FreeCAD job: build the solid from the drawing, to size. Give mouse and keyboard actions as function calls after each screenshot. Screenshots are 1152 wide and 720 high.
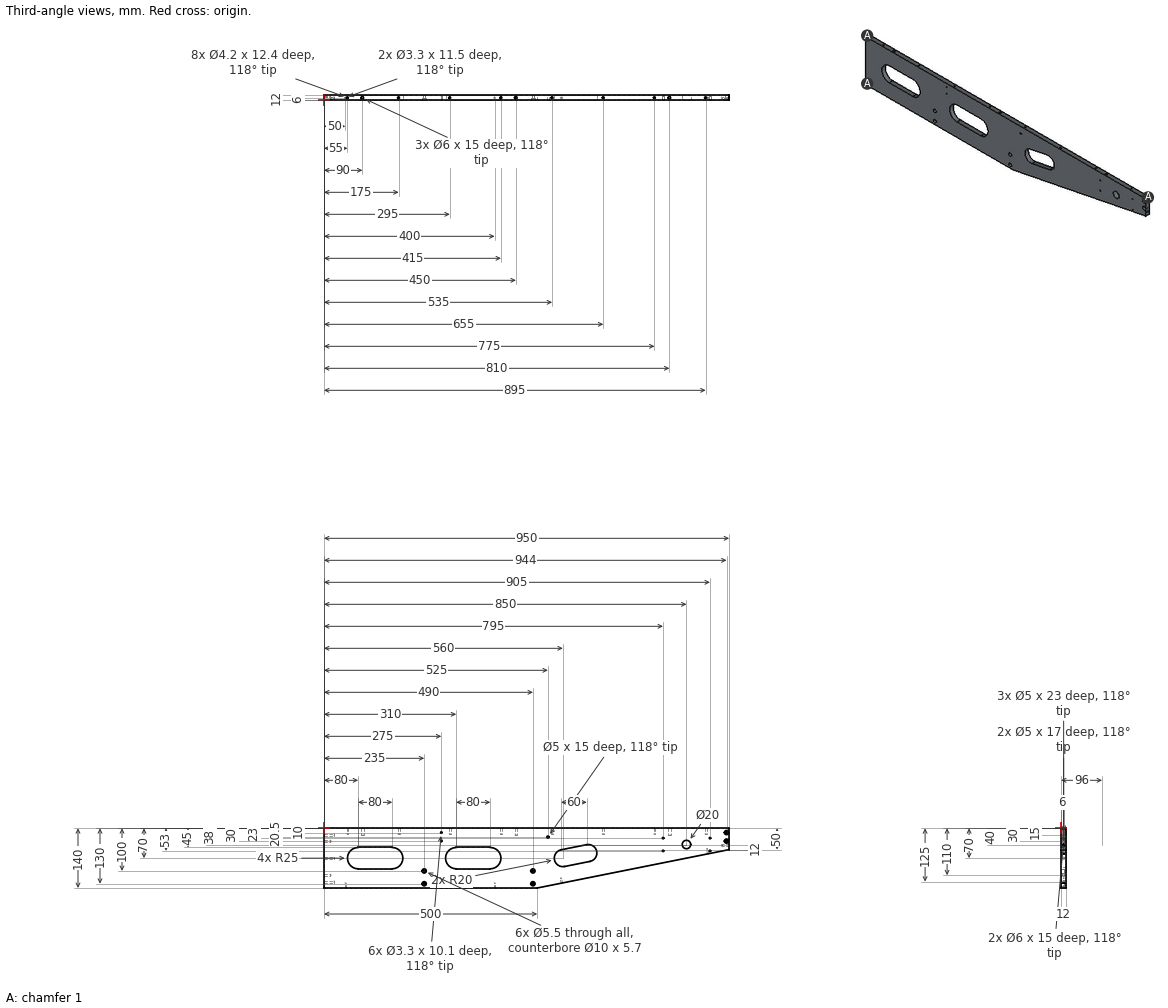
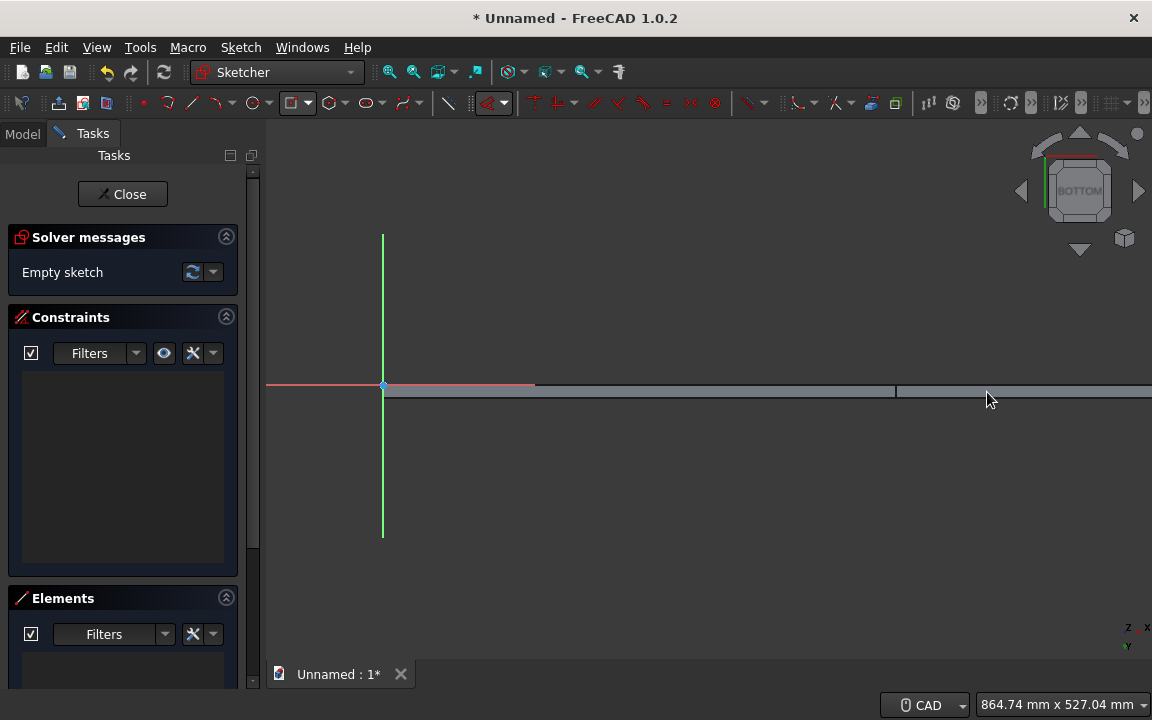
key(g)
key(c)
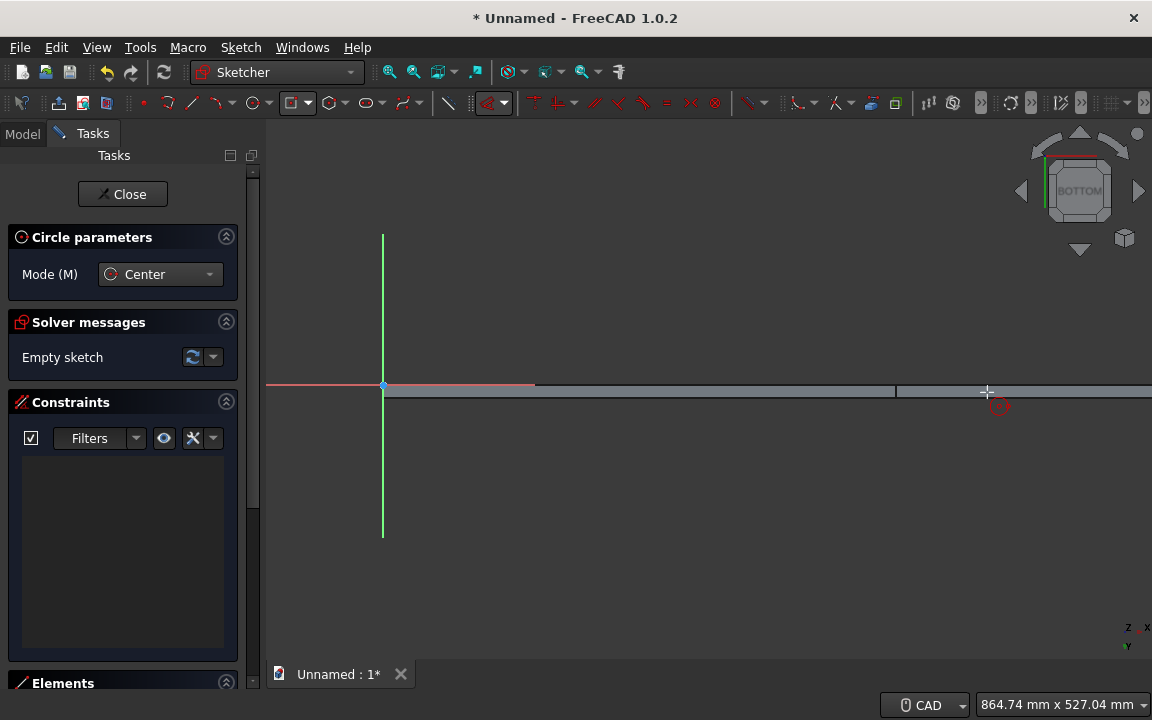
scroll(435, 392, up, 13)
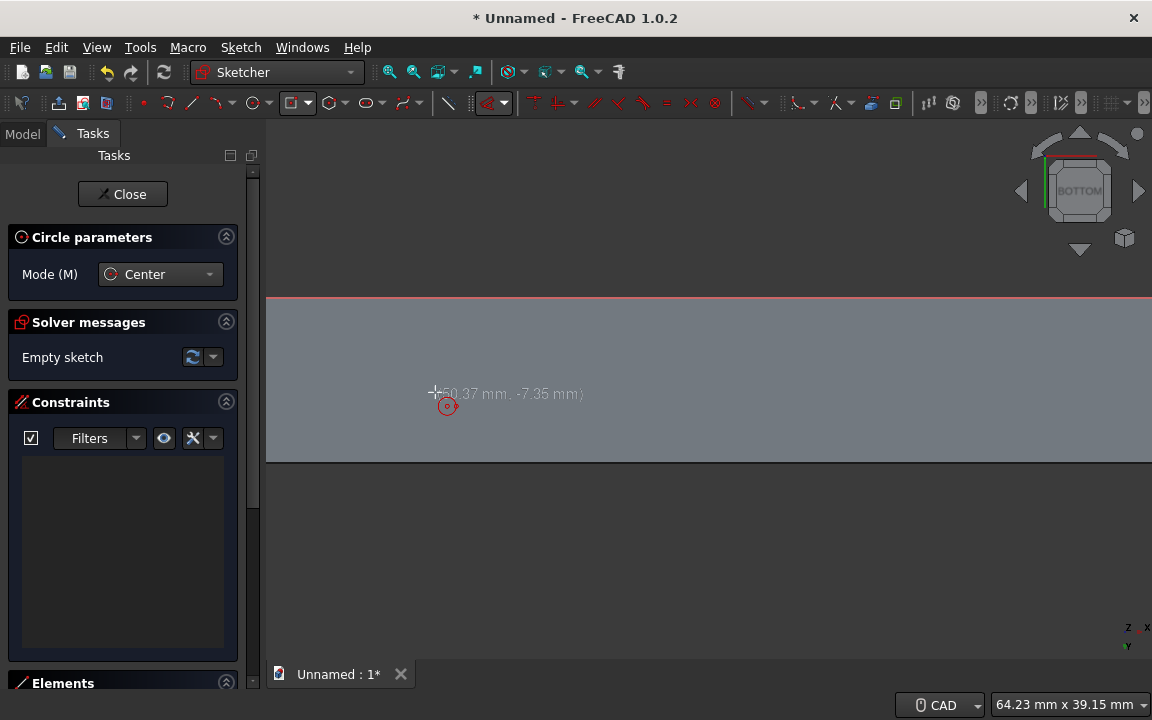
scroll(454, 393, down, 12)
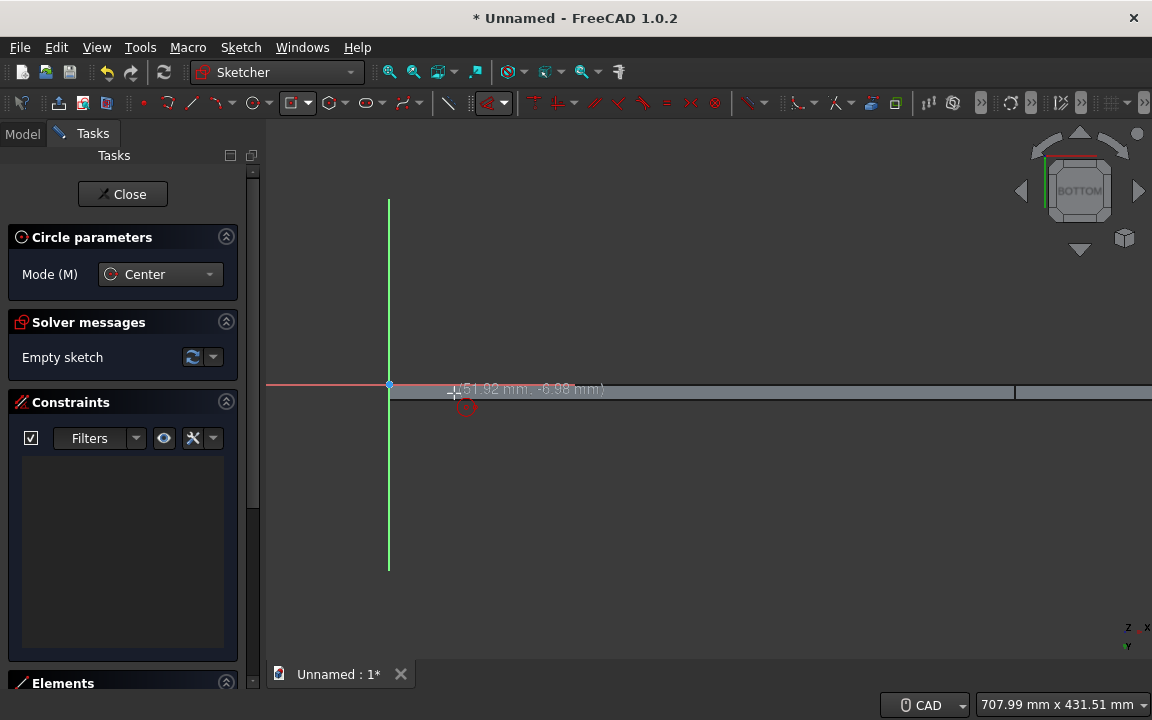
scroll(452, 392, up, 4)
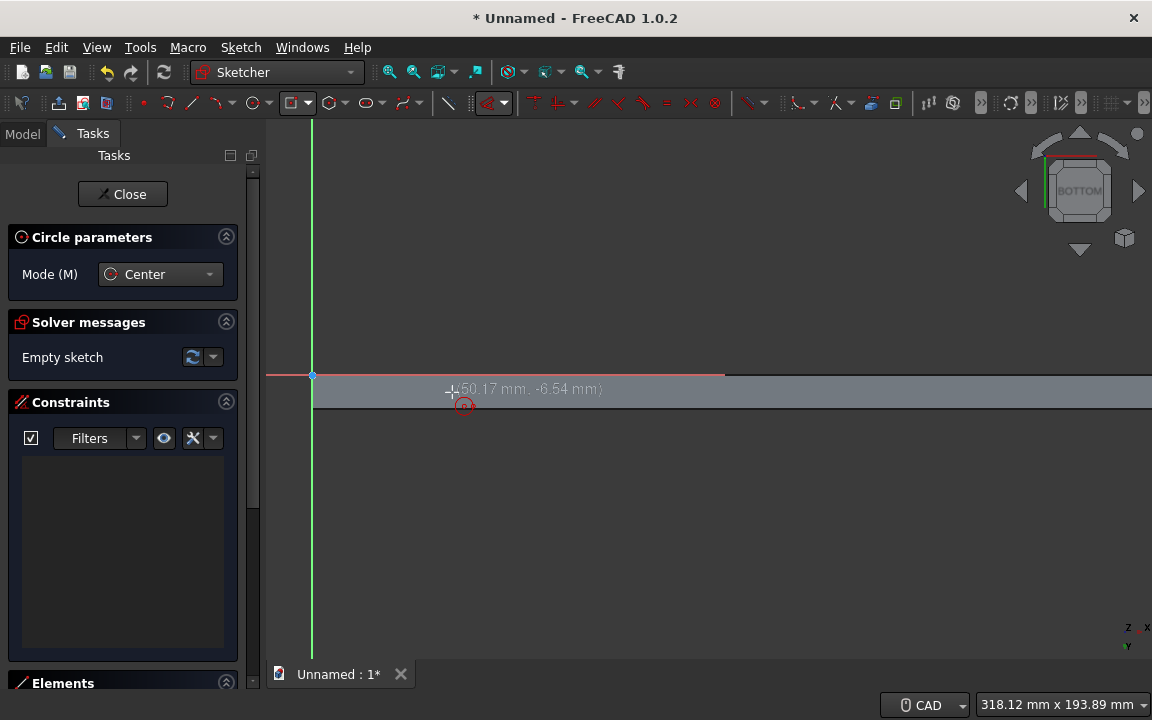
click(451, 392)
move(455, 395)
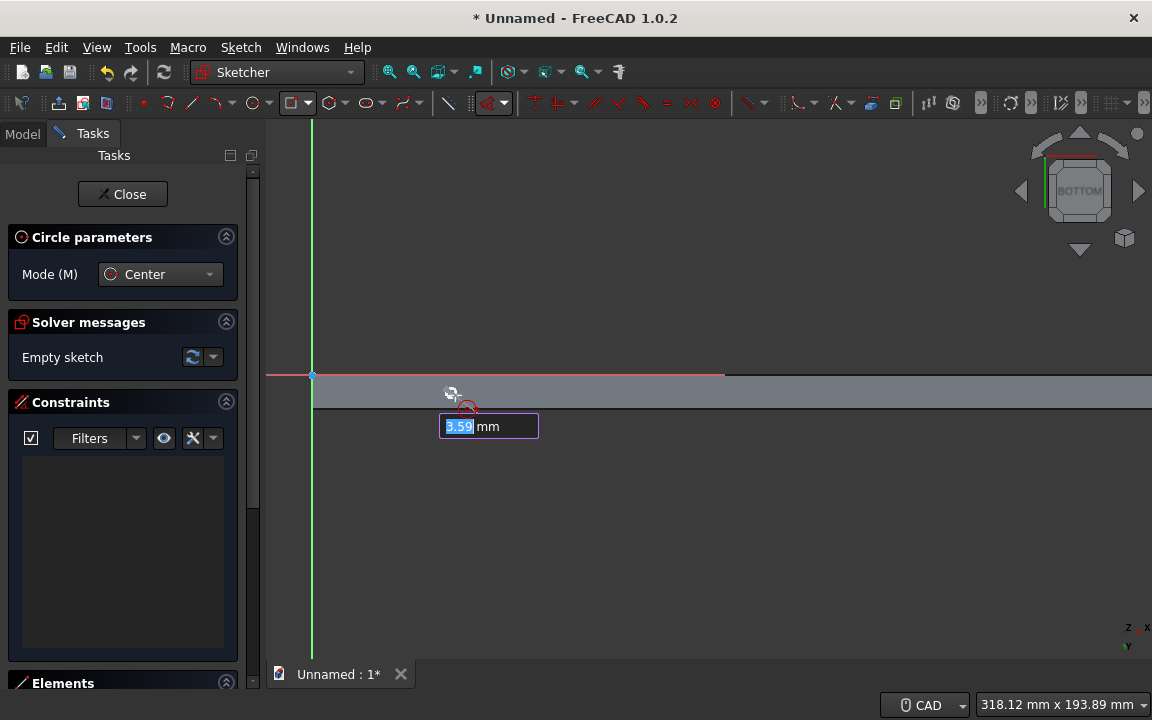
text(3.3)
key(Return)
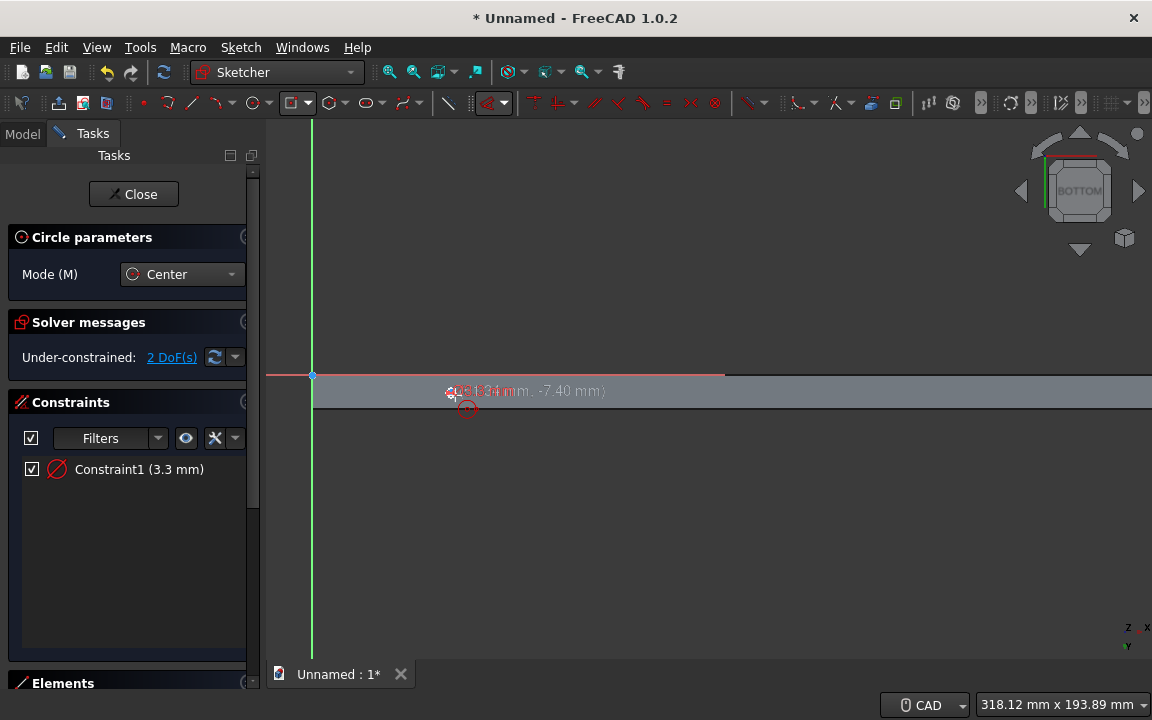
scroll(452, 391, down, 4)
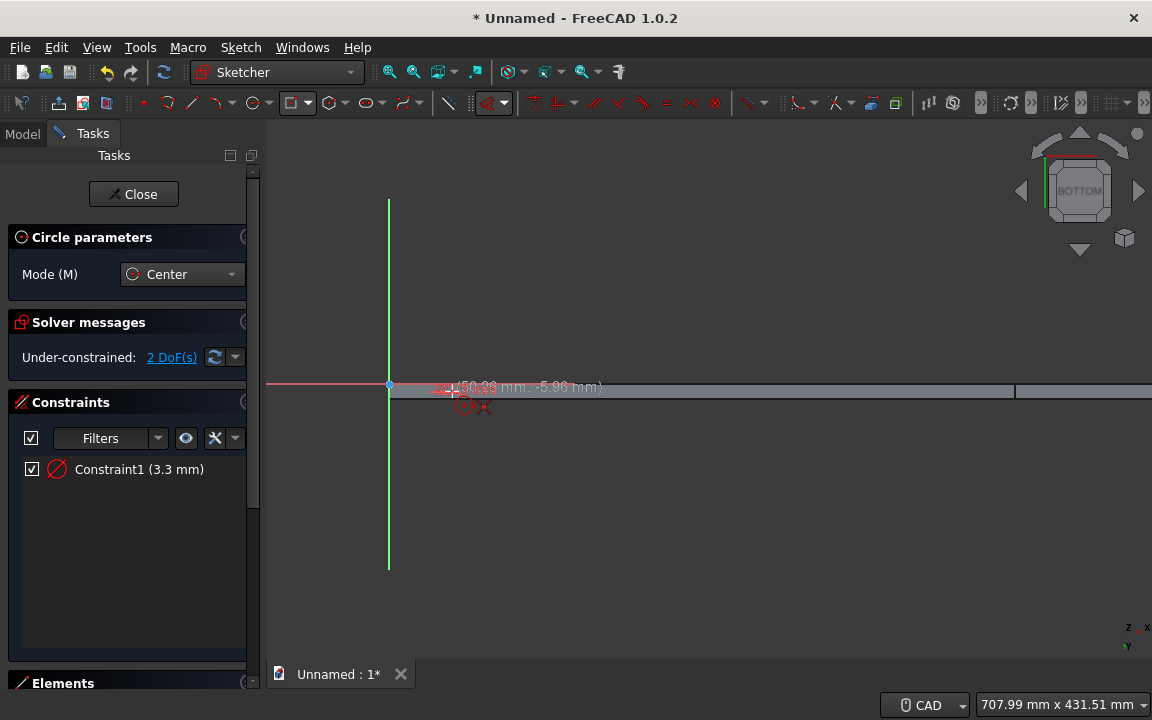
scroll(890, 392, up, 12)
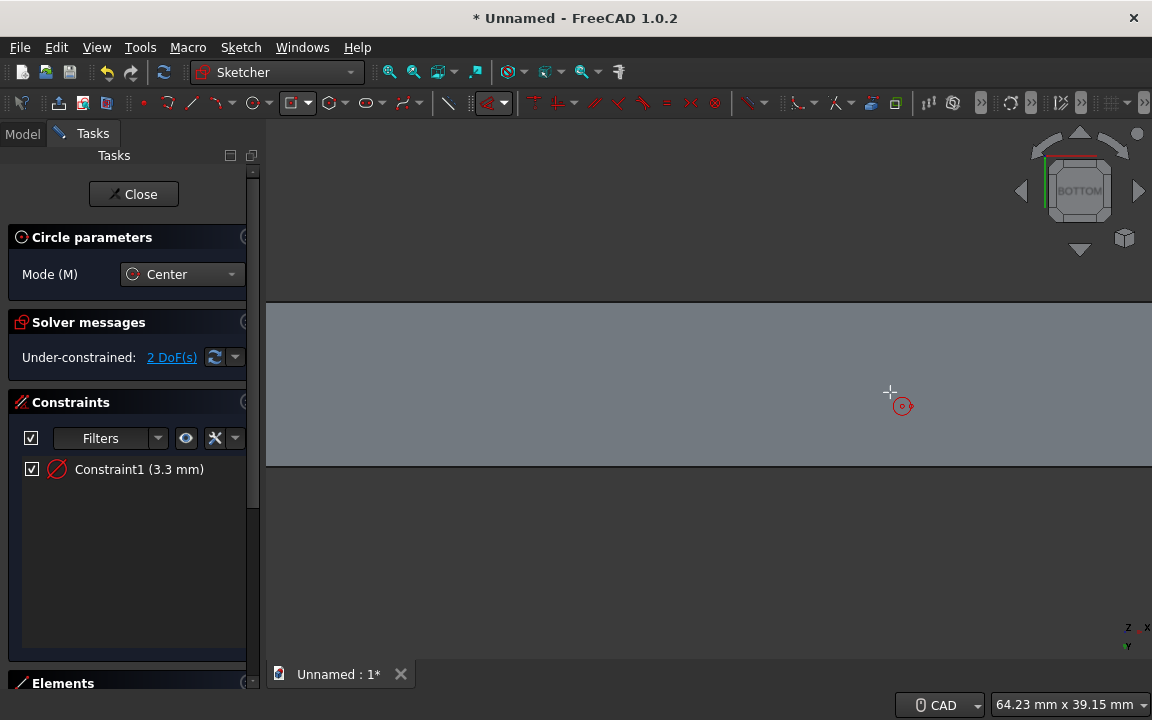
scroll(891, 392, down, 12)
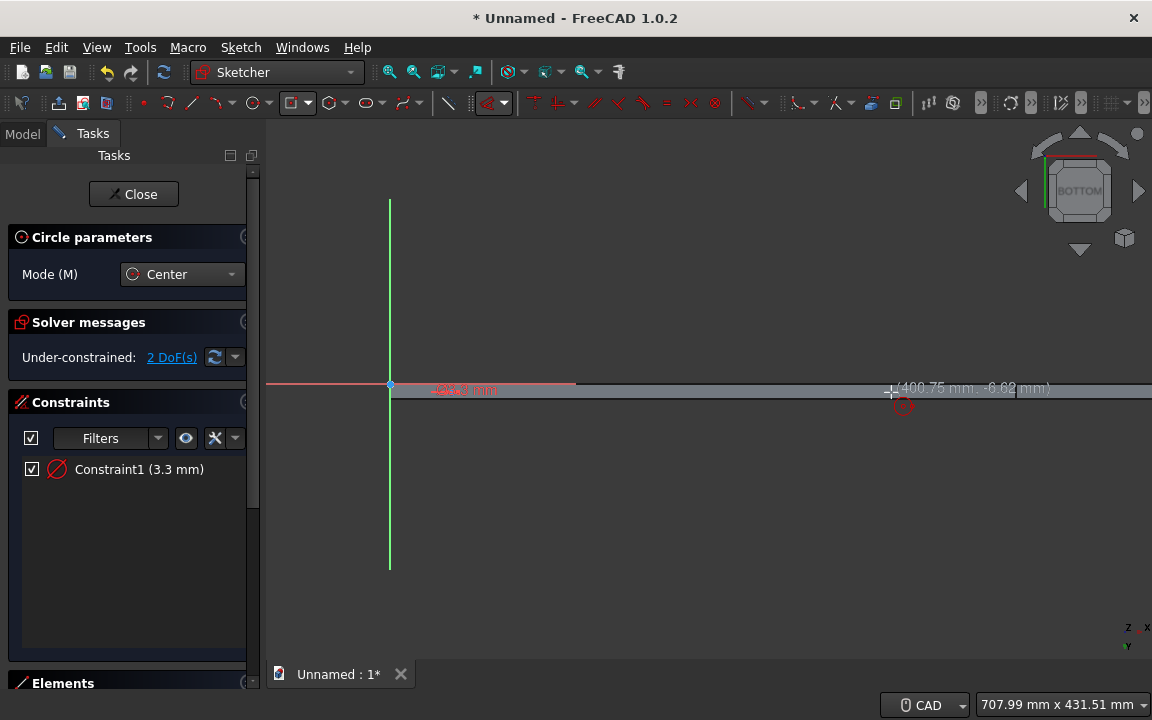
scroll(891, 392, up, 4)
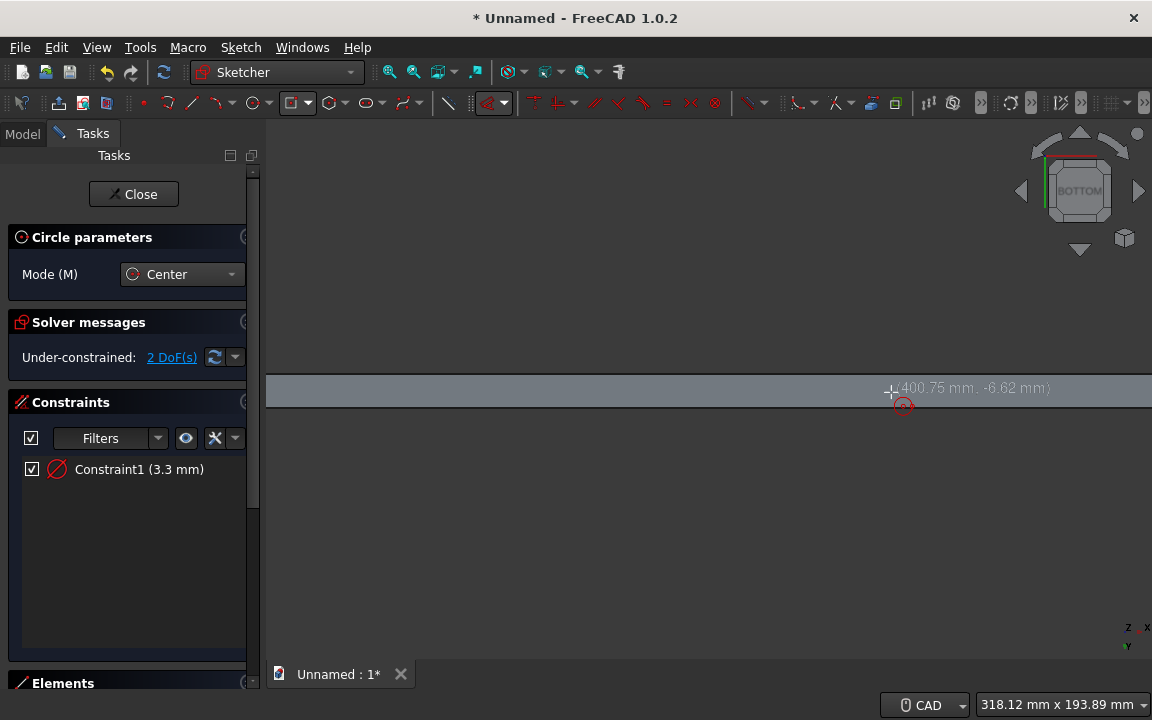
click(889, 391)
move(893, 394)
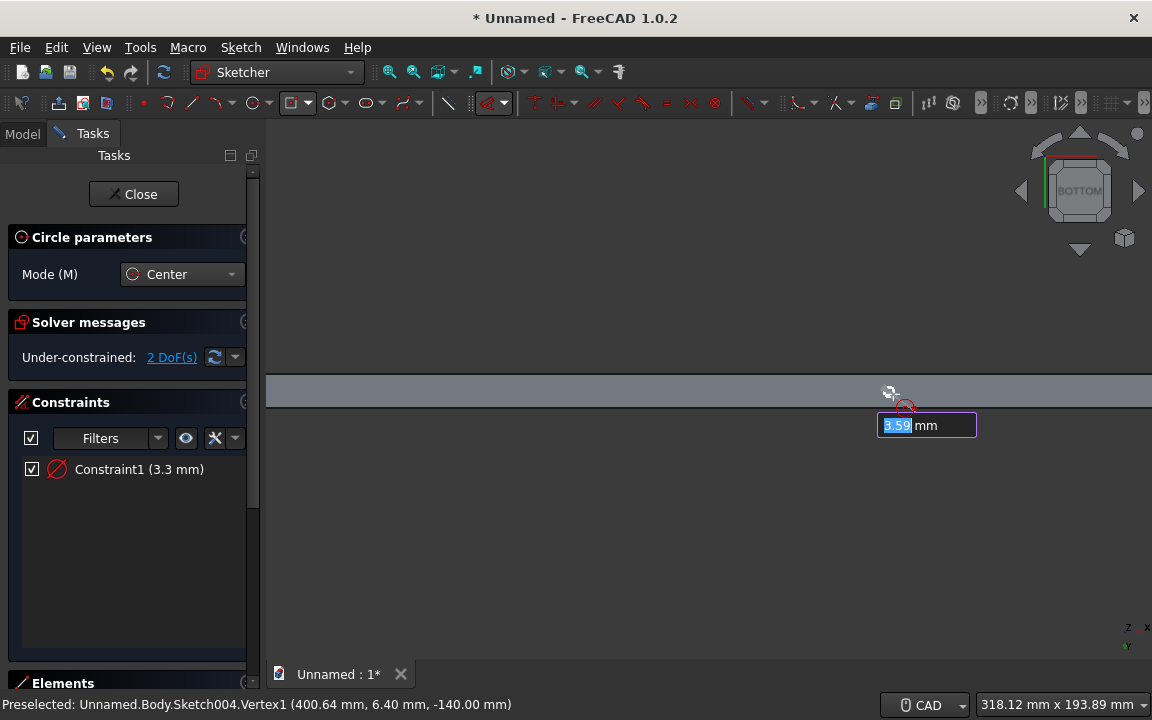
text(3.3)
key(Return)
key(Escape)